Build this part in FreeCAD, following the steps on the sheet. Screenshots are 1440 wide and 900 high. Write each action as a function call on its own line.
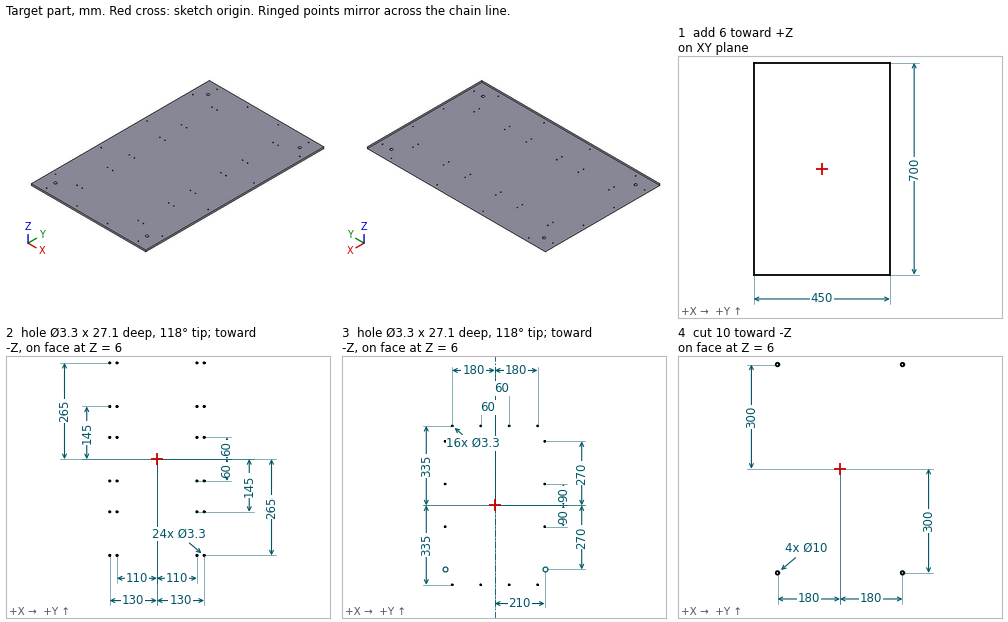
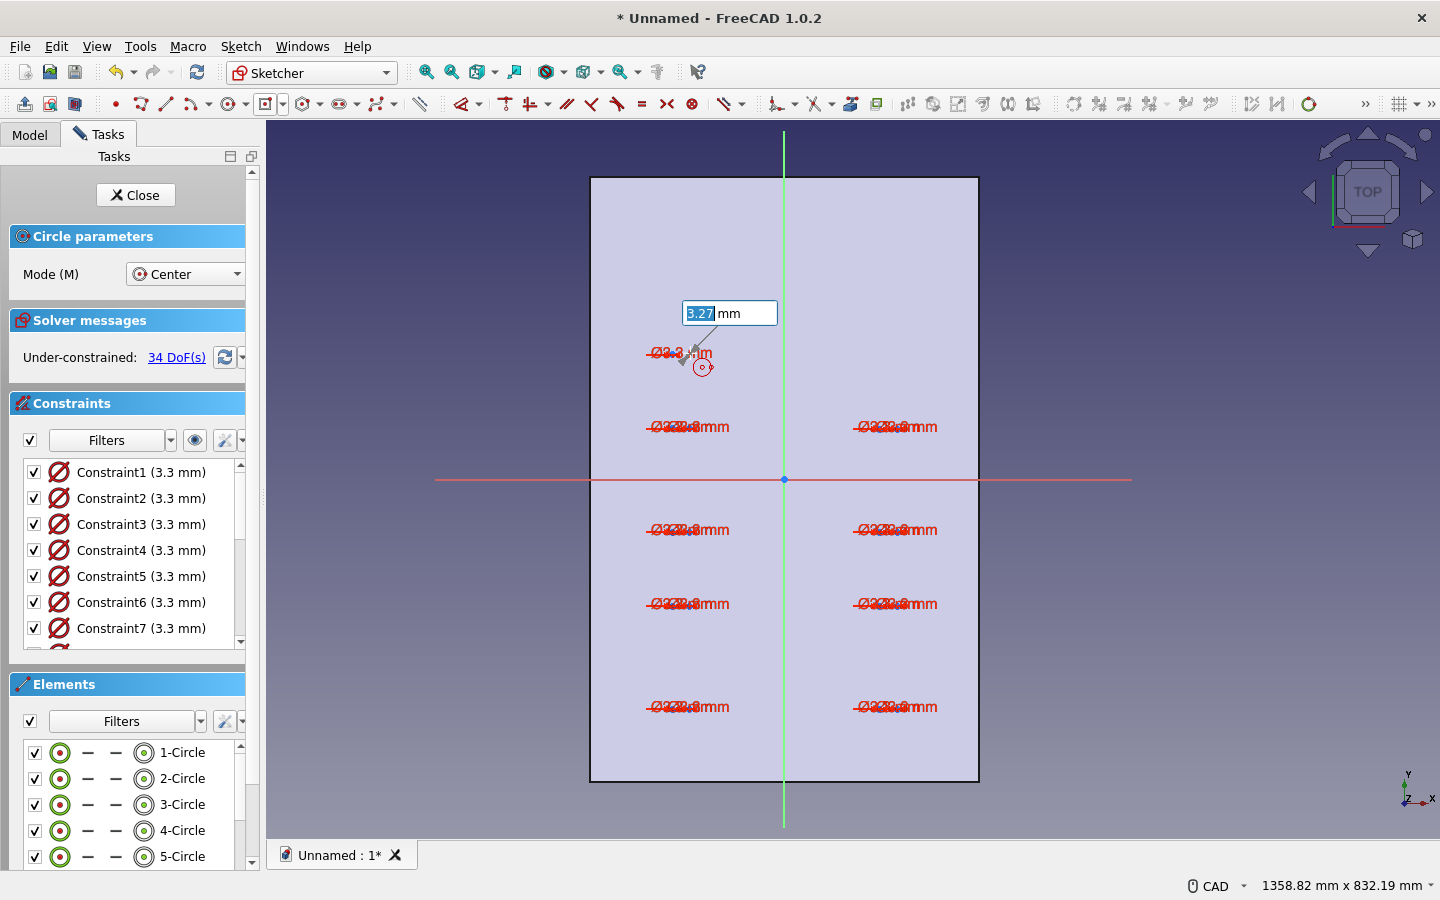
text(3.3)
key(Return)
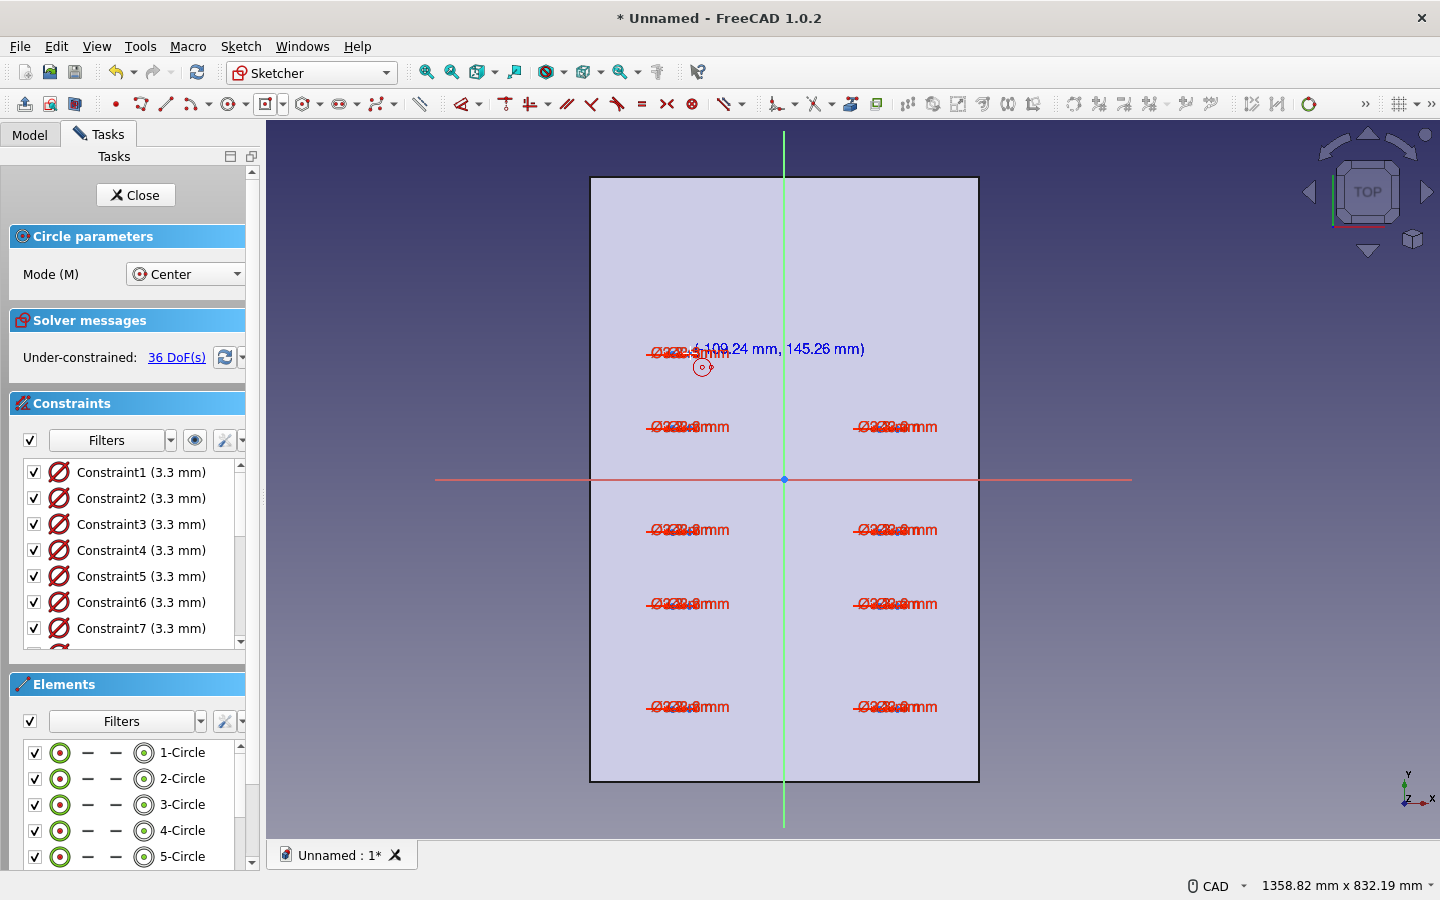
scroll(672, 251, up, 14)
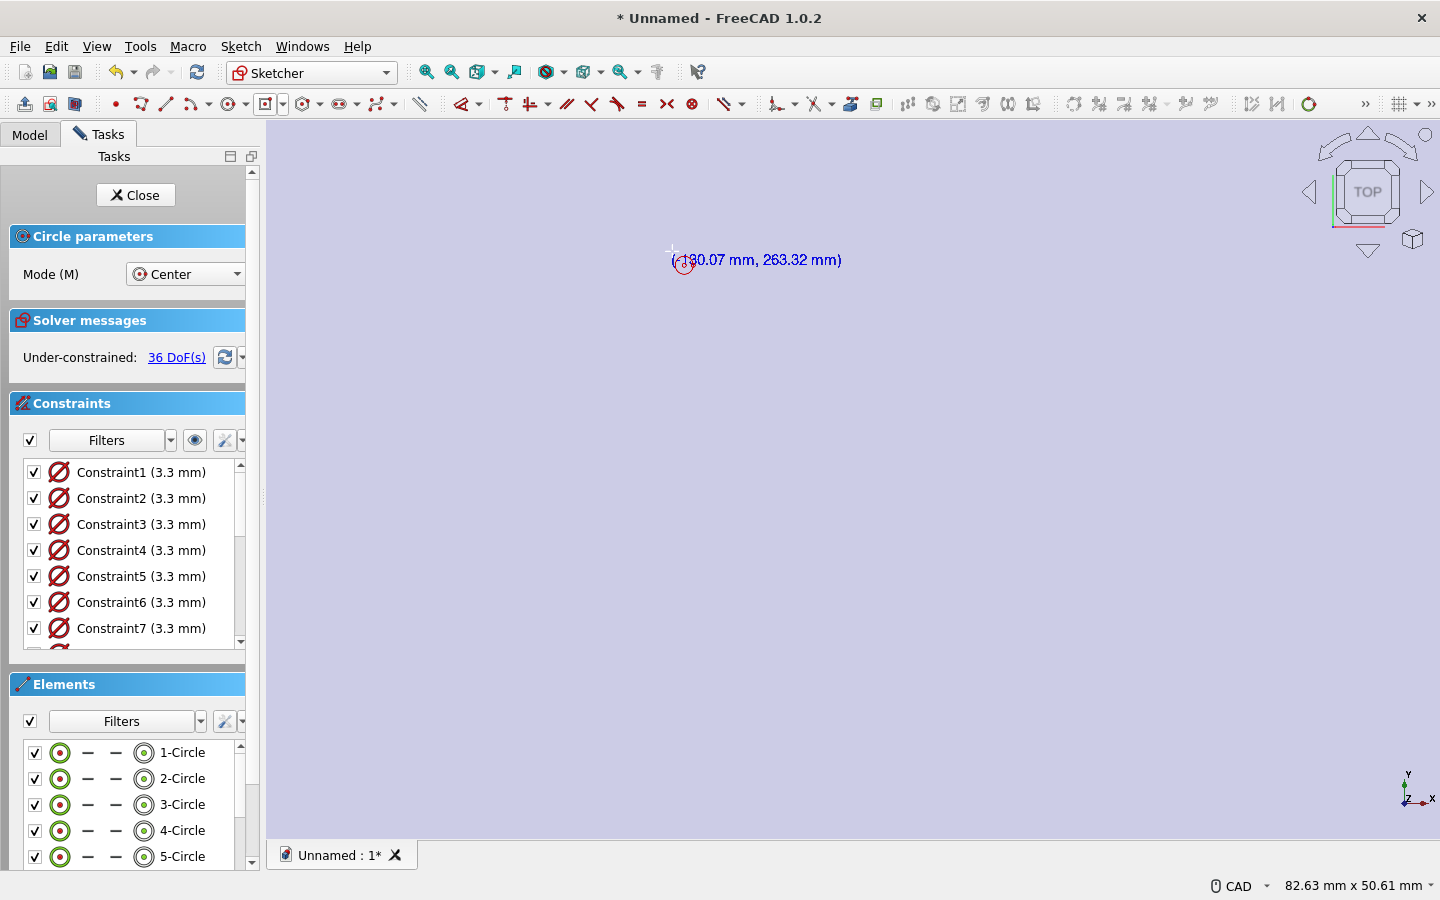
scroll(672, 251, down, 14)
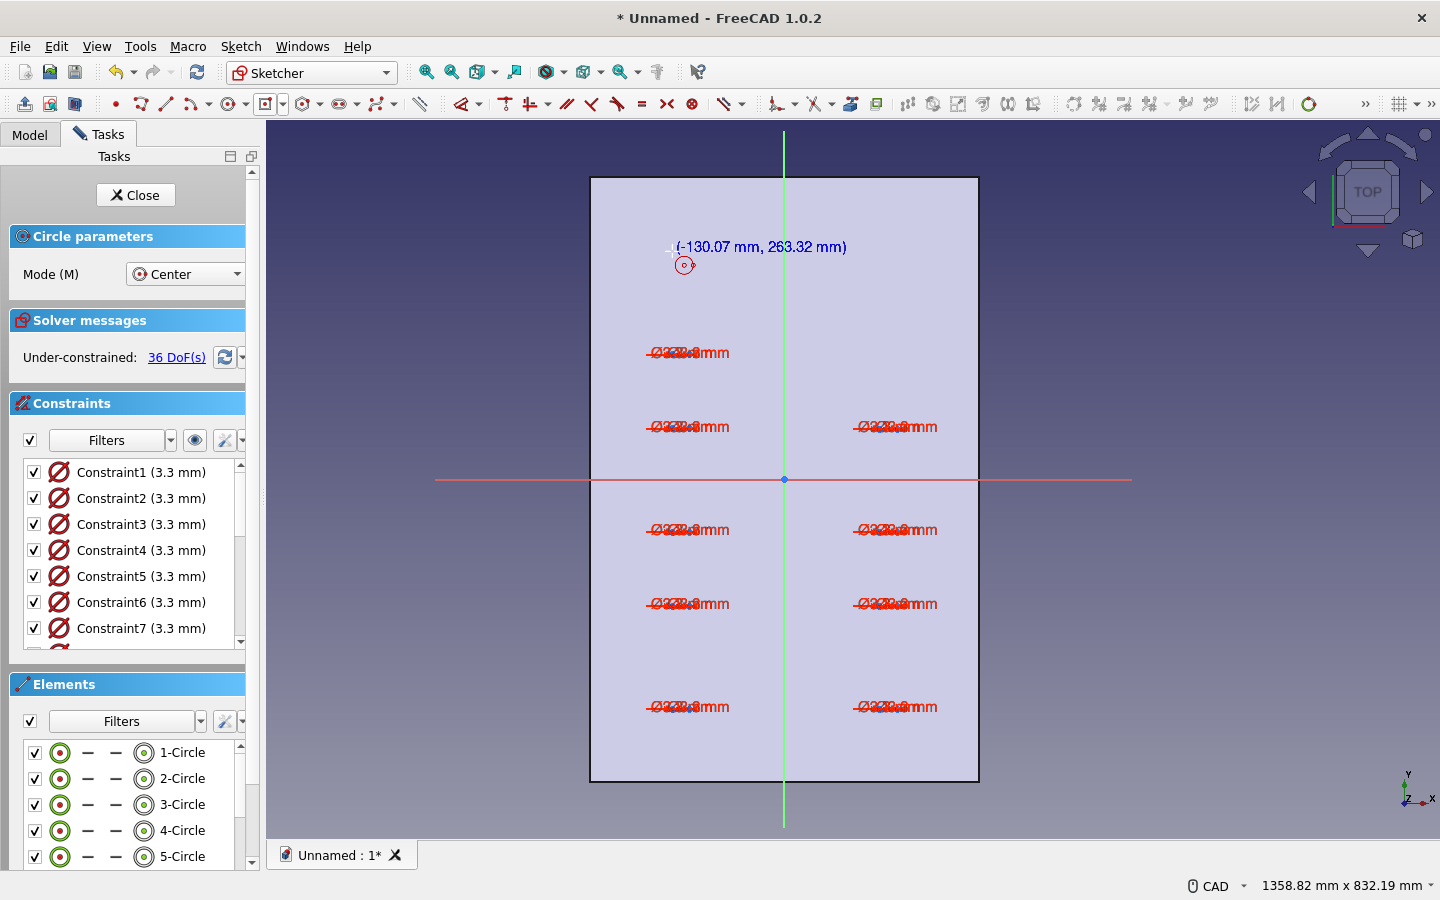
click(672, 251)
move(673, 250)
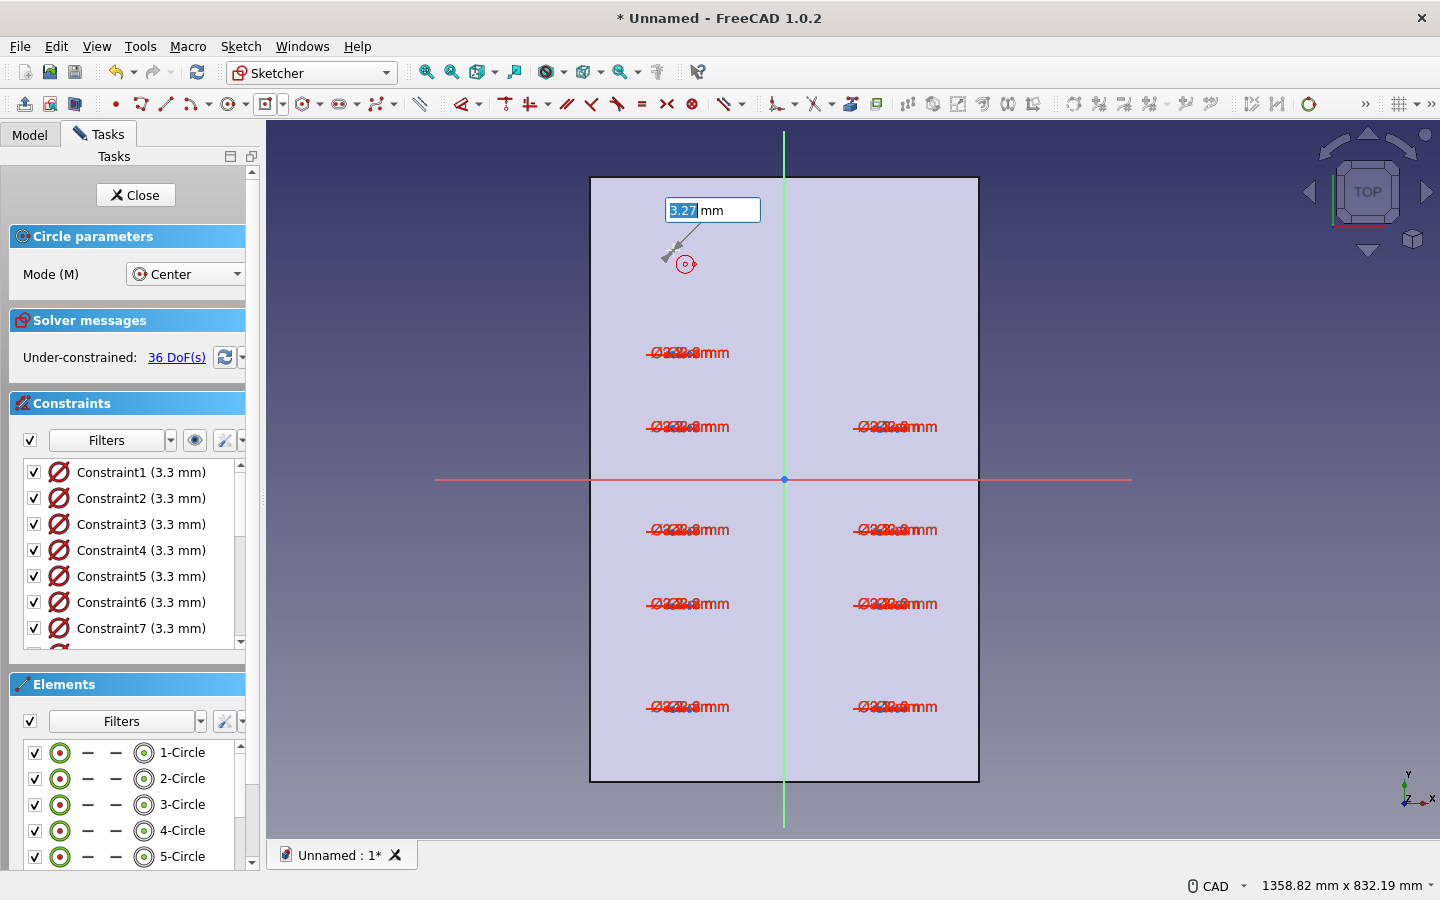
text(3.3)
key(Return)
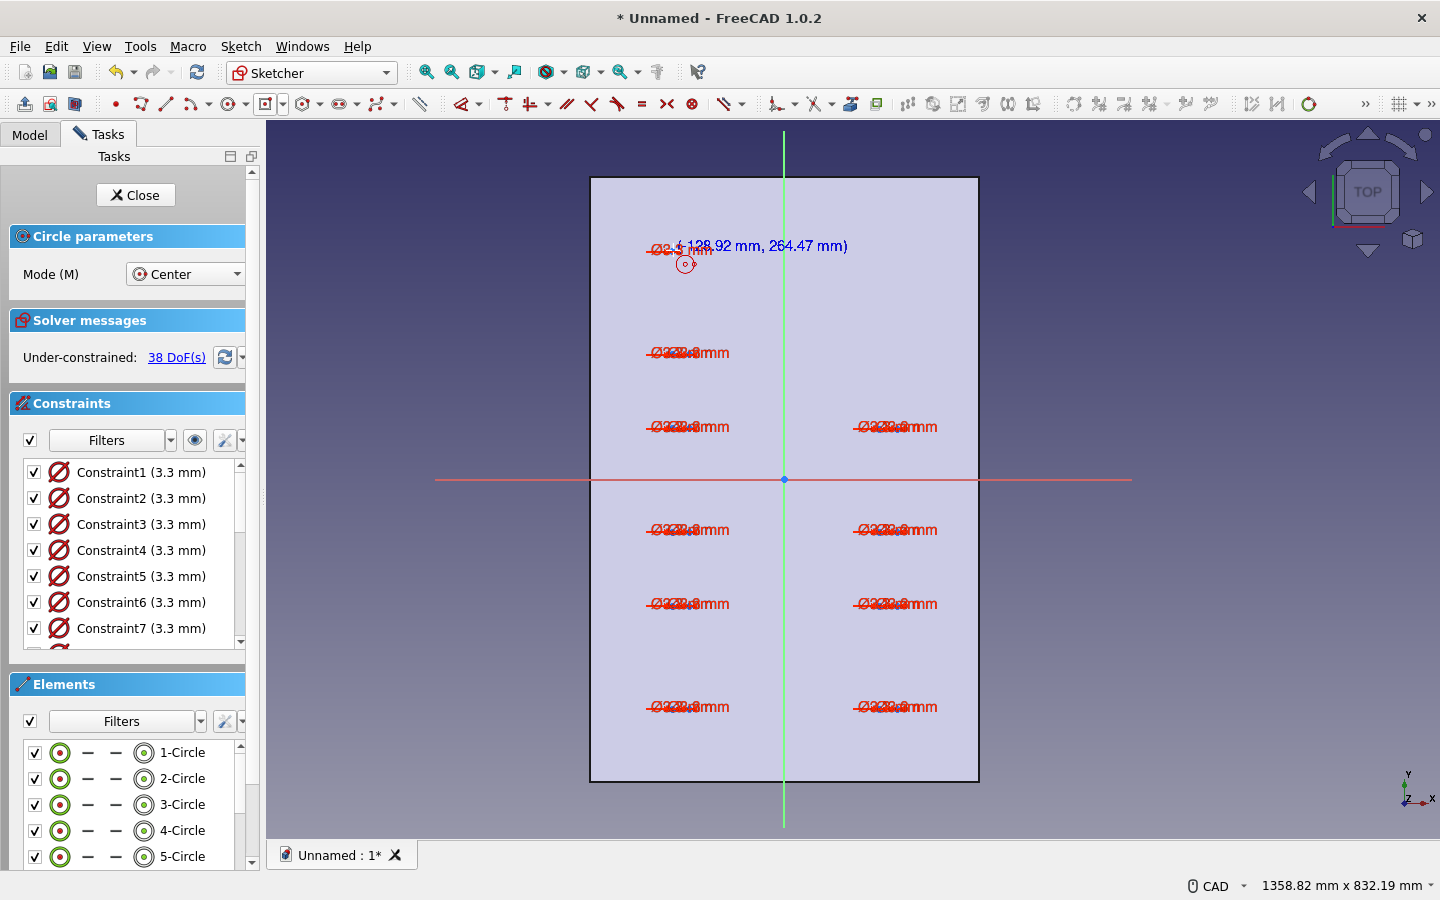
scroll(689, 251, up, 14)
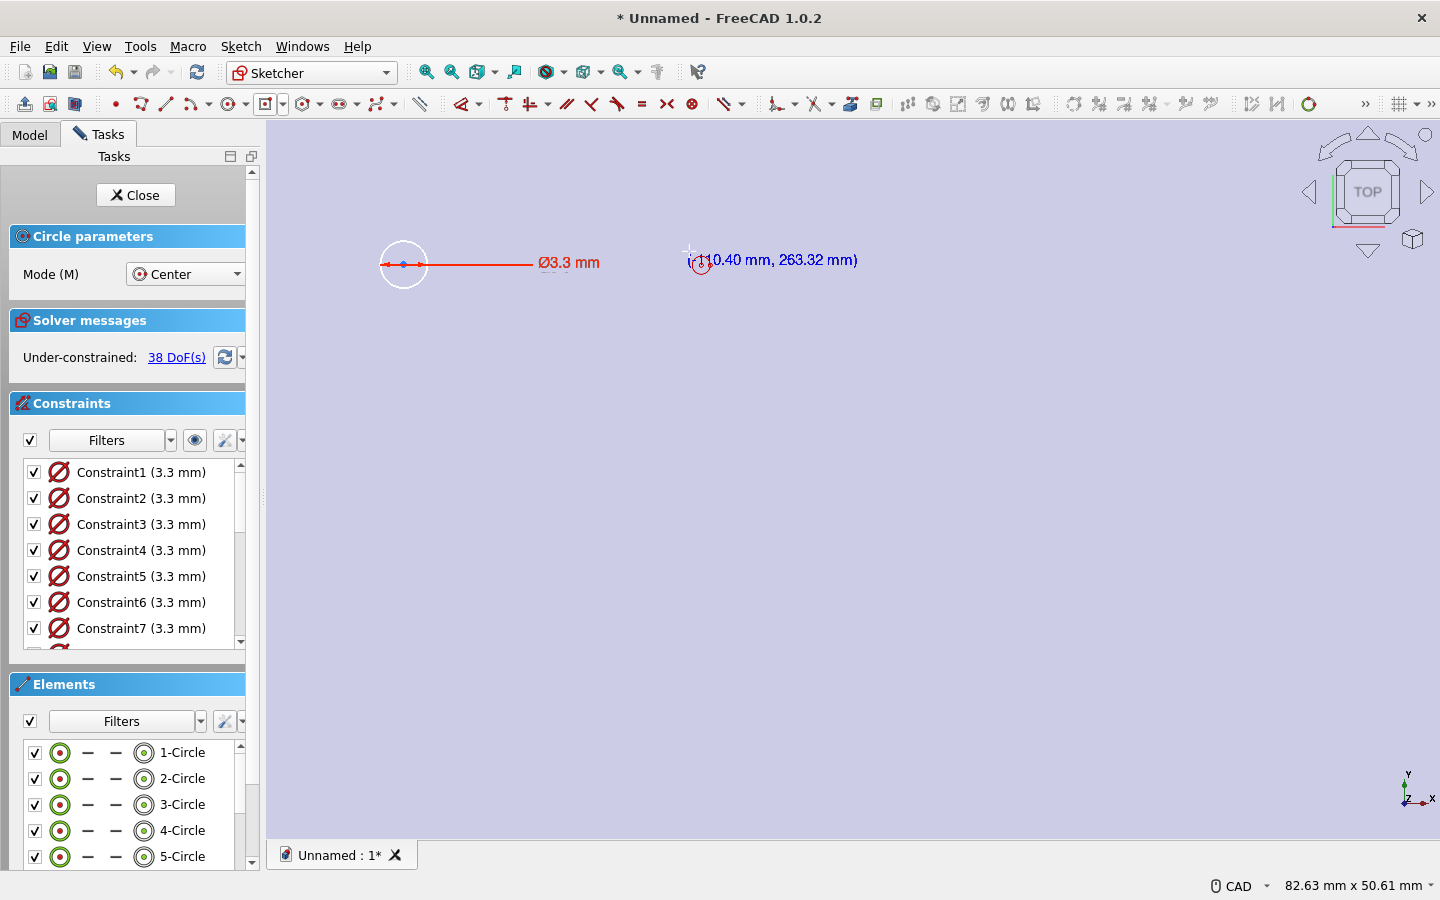
scroll(689, 251, down, 14)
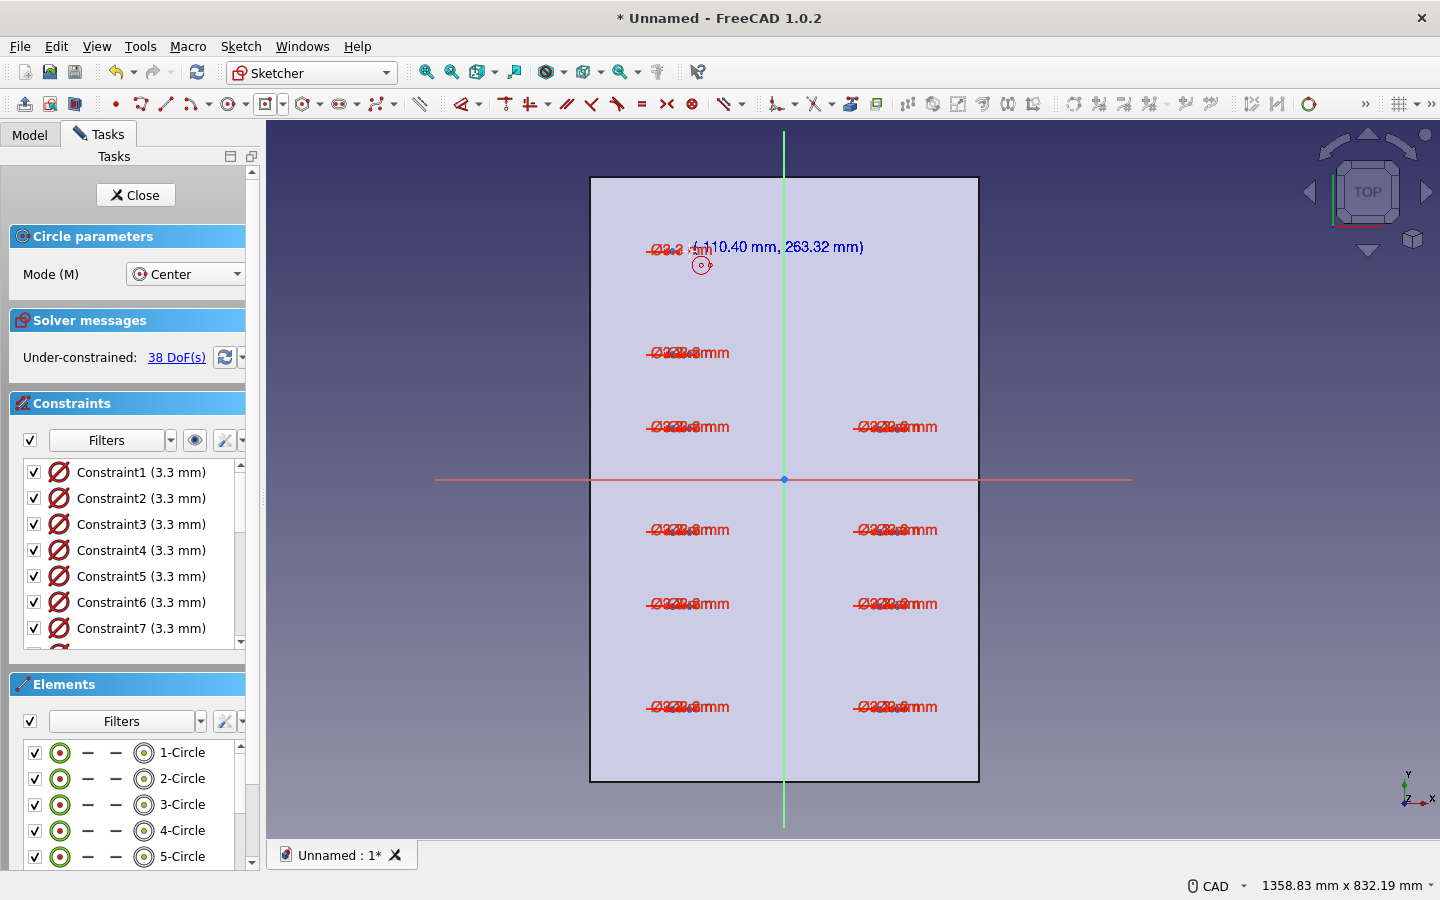
click(689, 251)
move(690, 250)